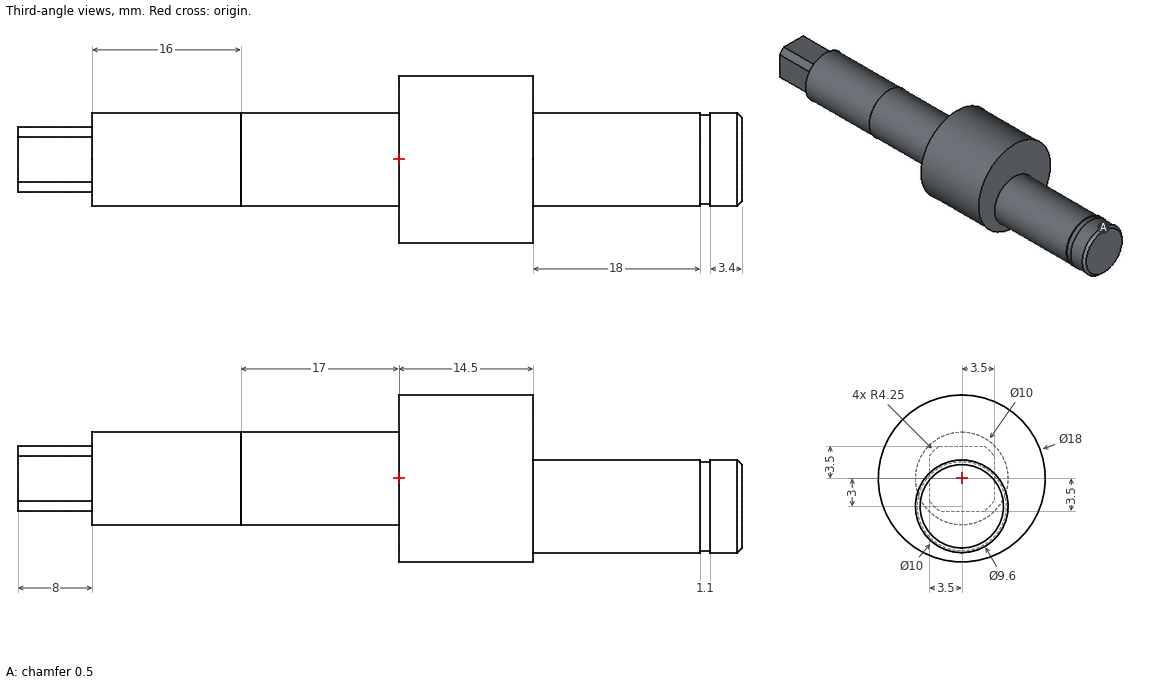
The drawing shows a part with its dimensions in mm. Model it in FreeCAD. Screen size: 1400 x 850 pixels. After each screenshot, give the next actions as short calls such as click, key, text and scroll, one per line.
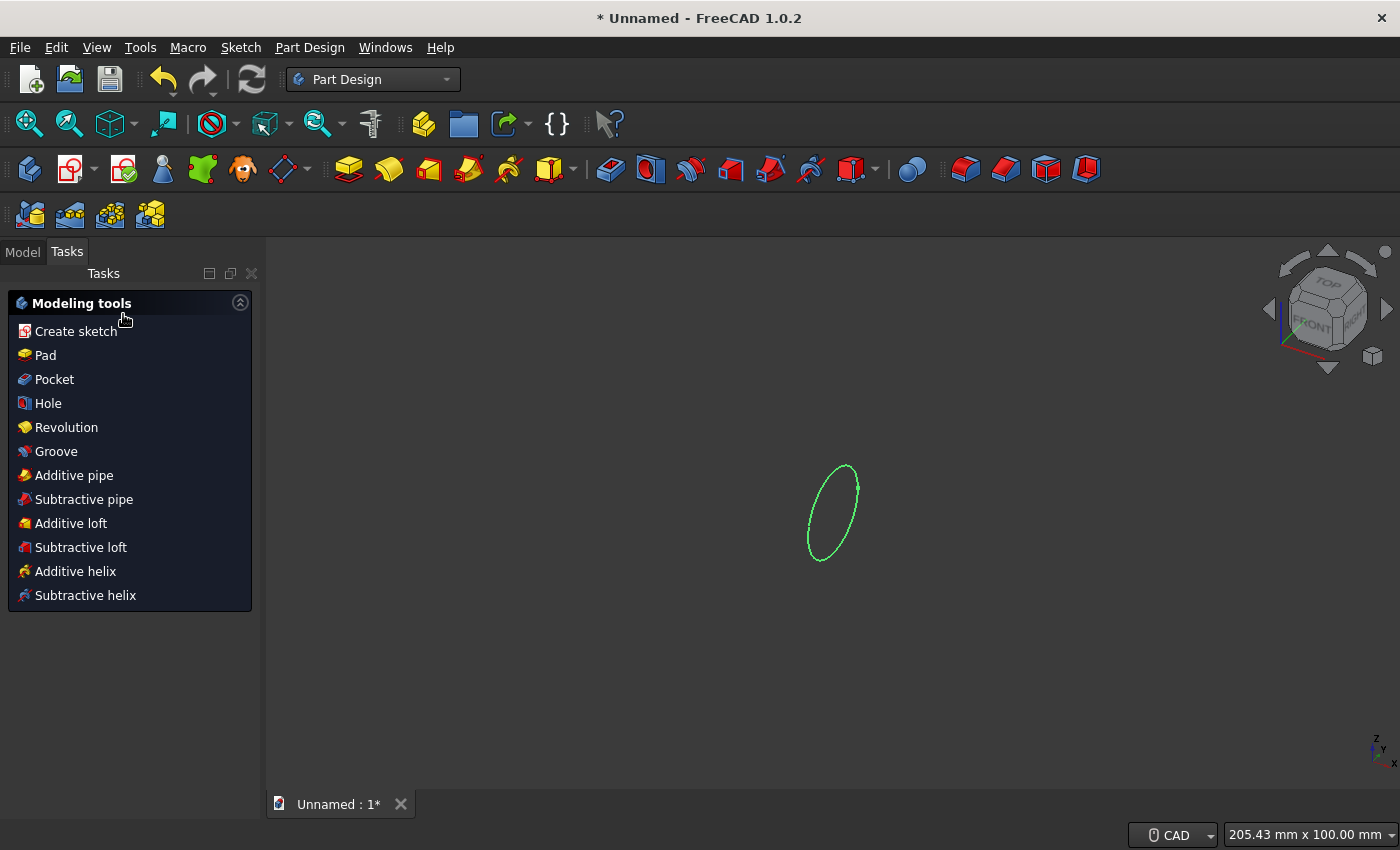
click(350, 170)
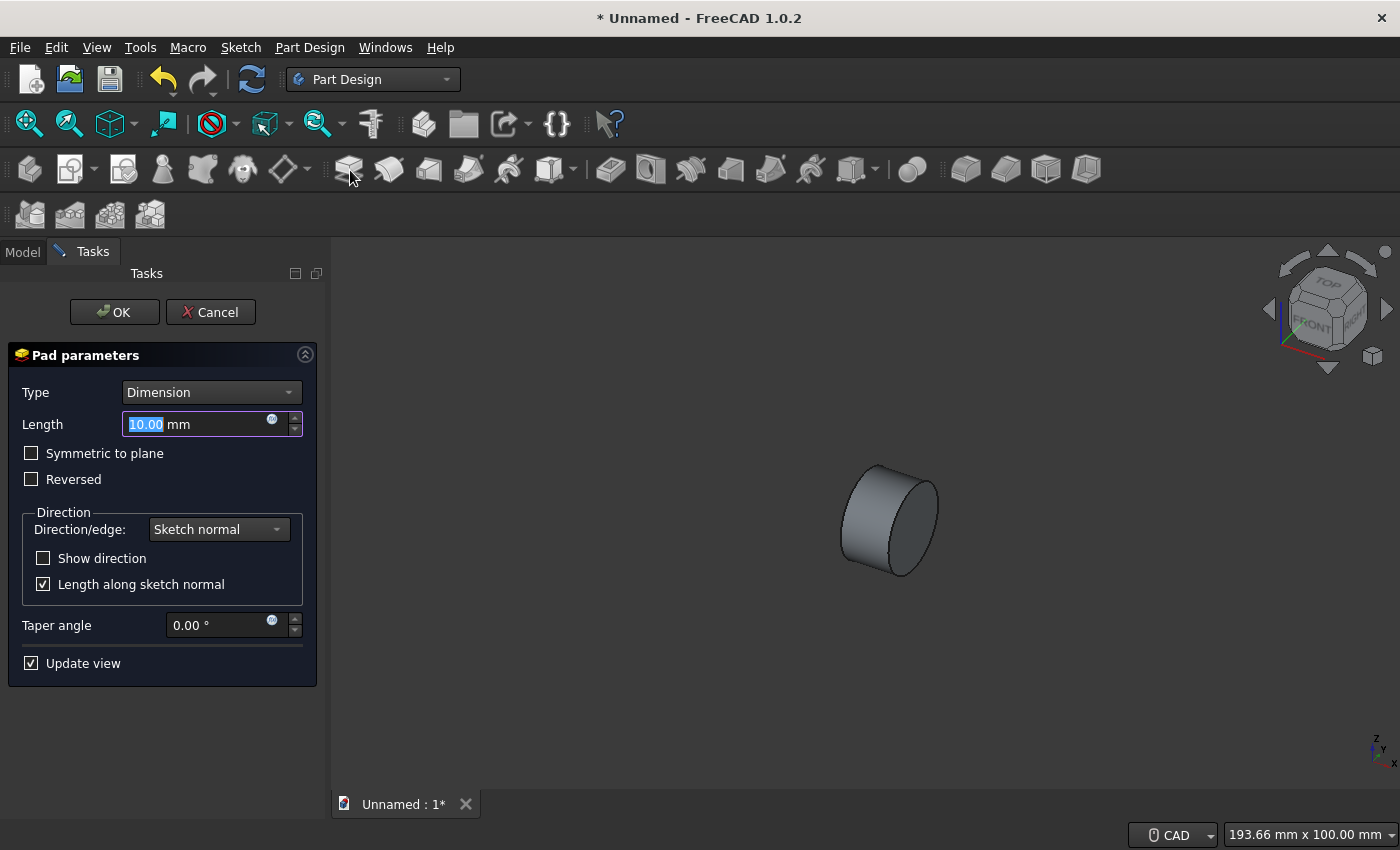
text(14.5)
key(Tab)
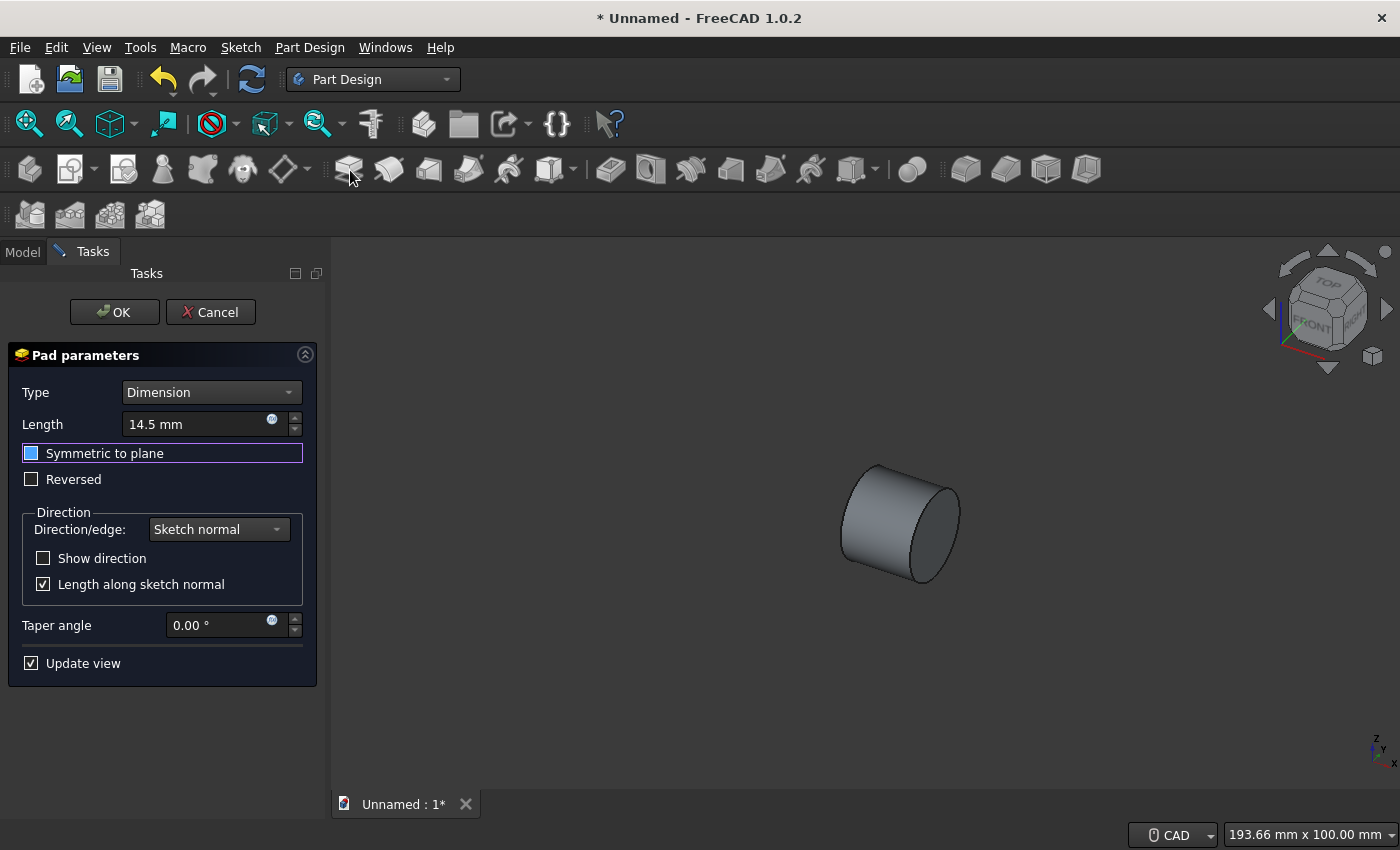
click(115, 312)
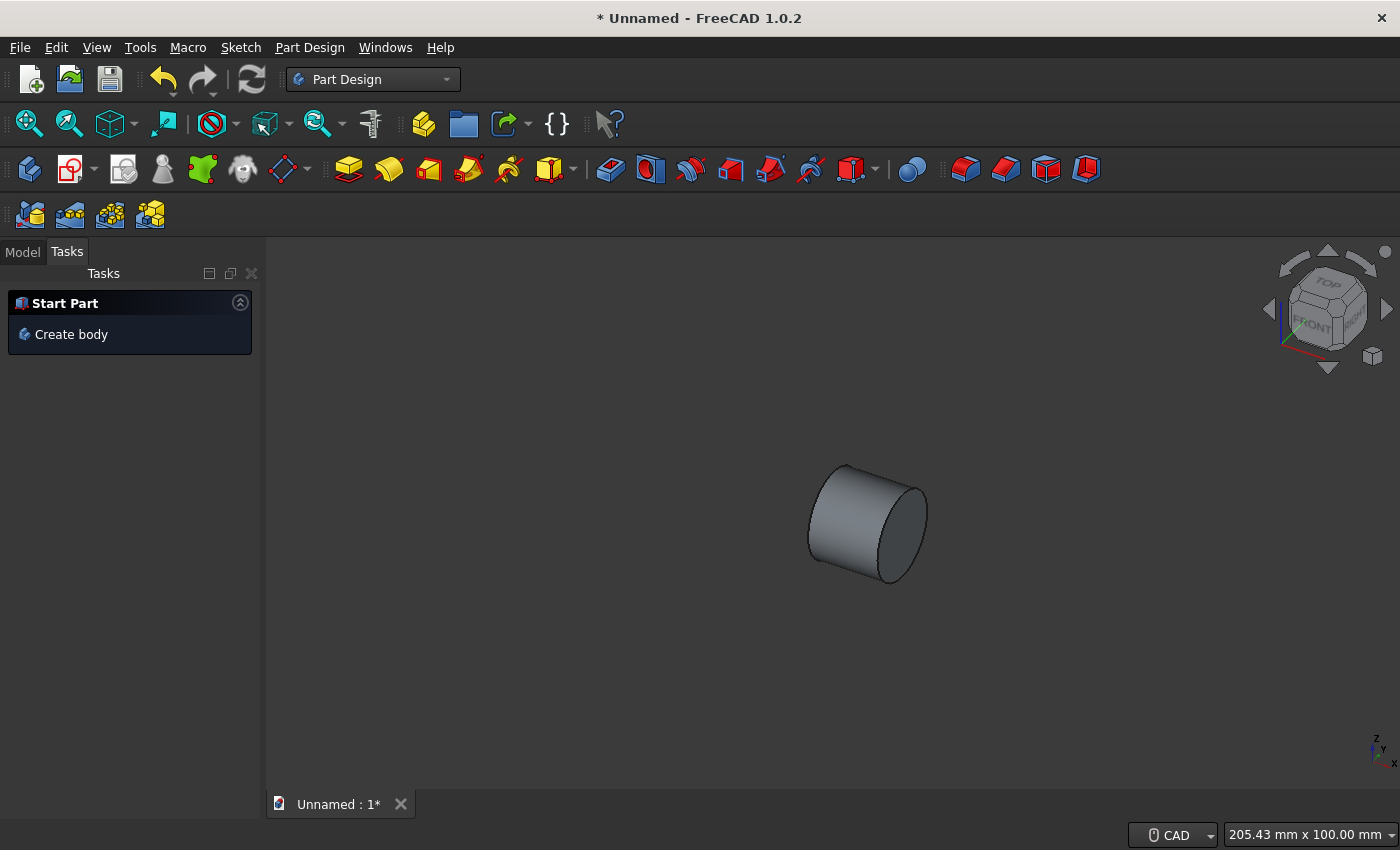
click(30, 124)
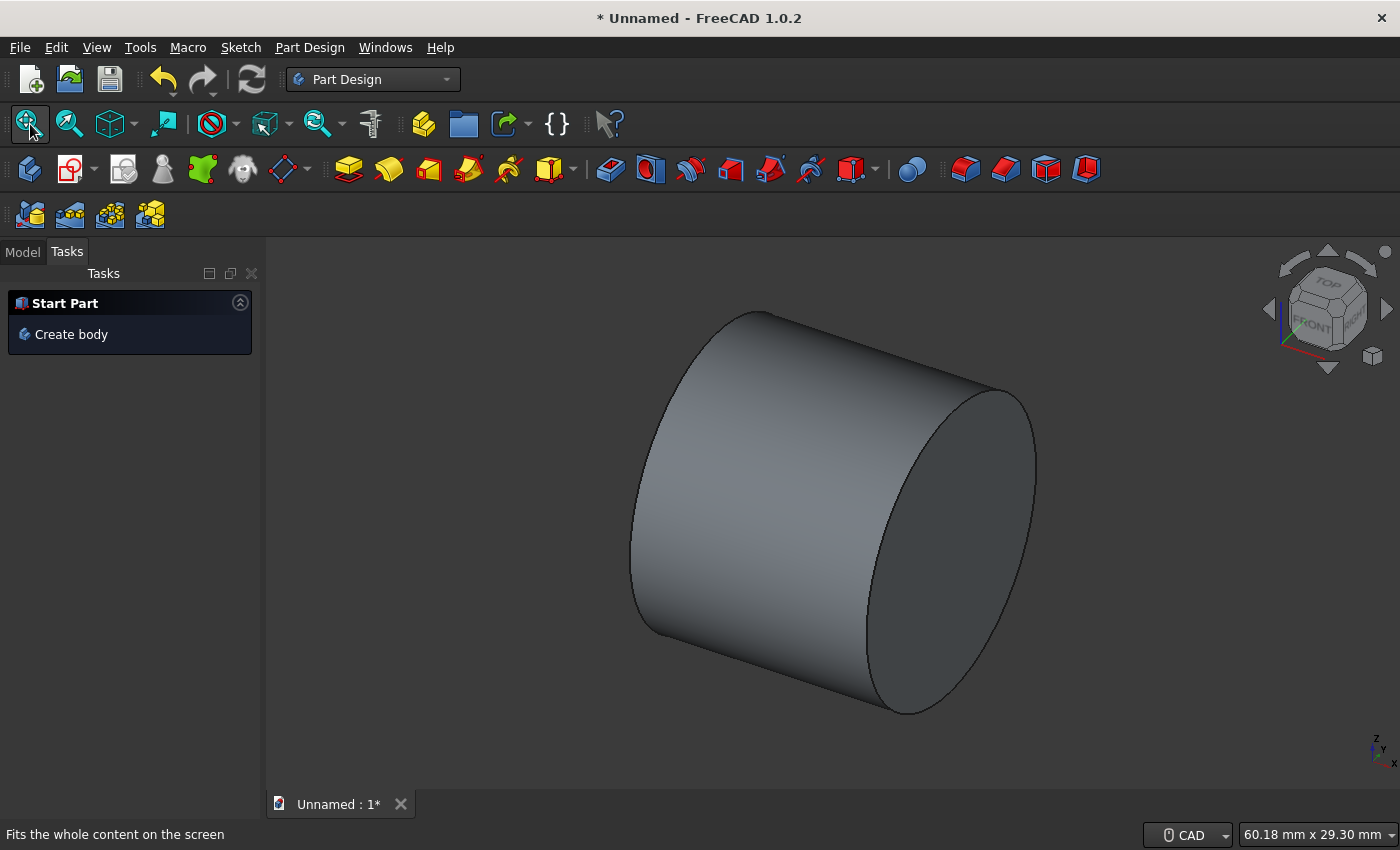
click(951, 551)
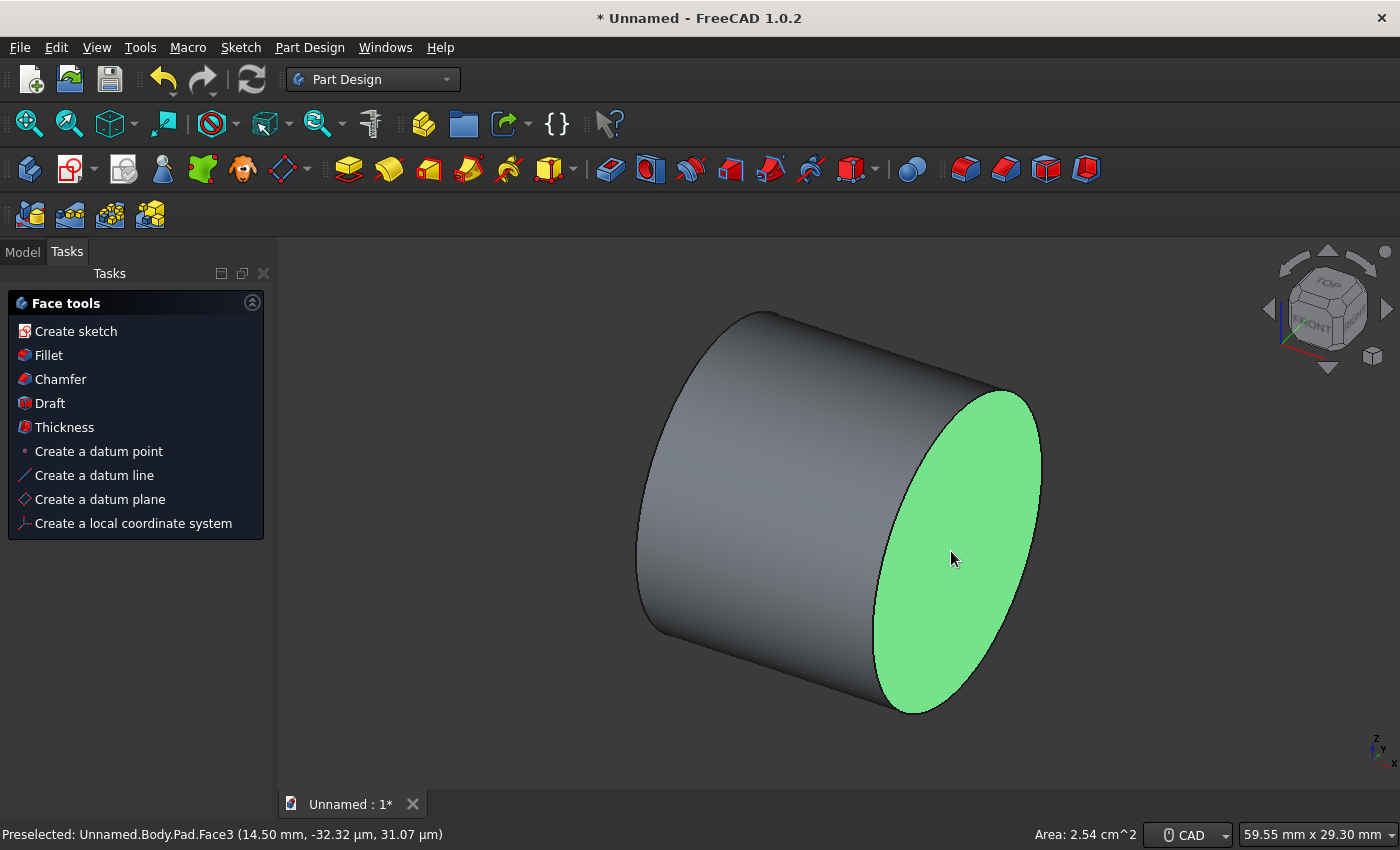
click(70, 170)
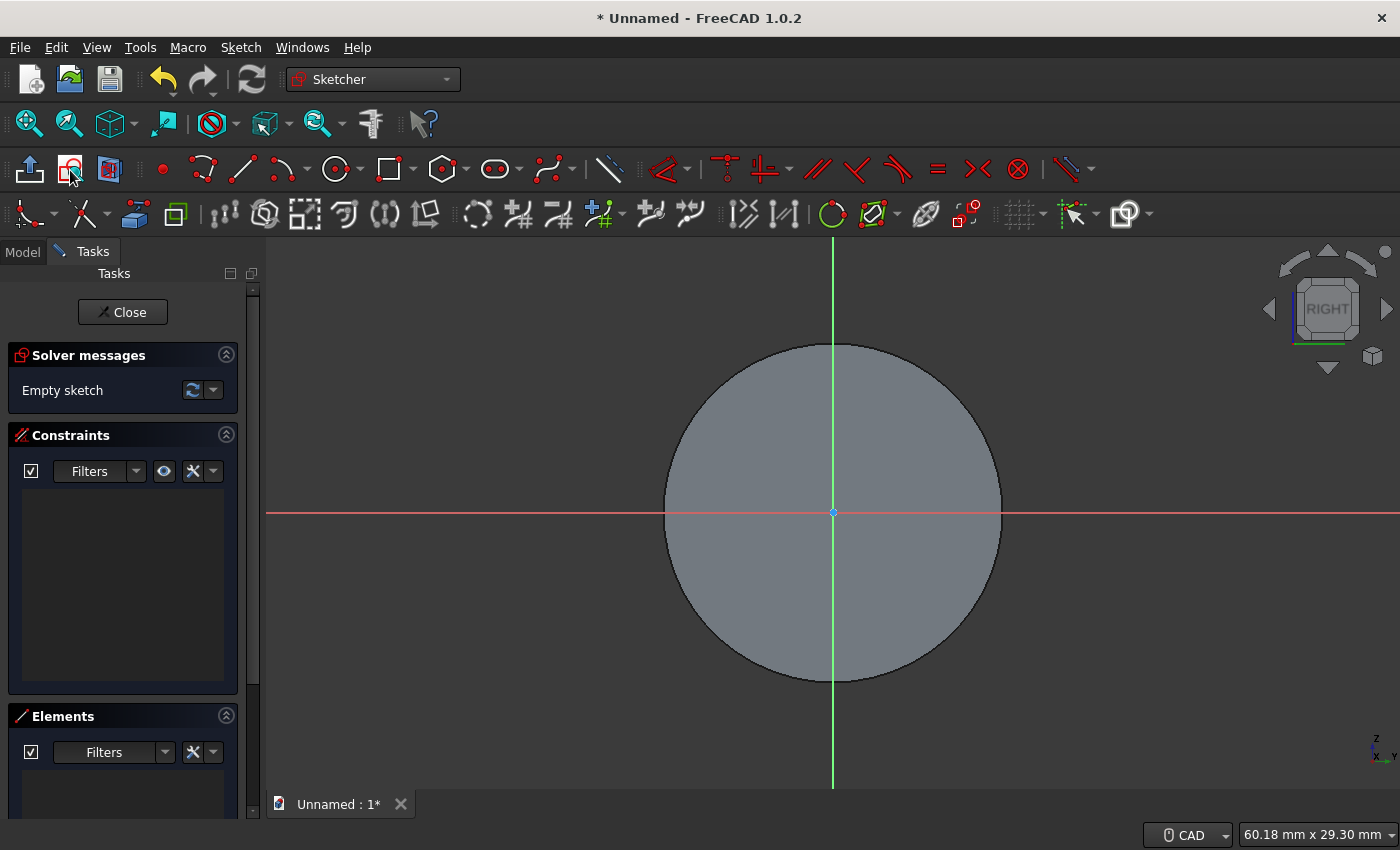
scroll(916, 638, up, 3)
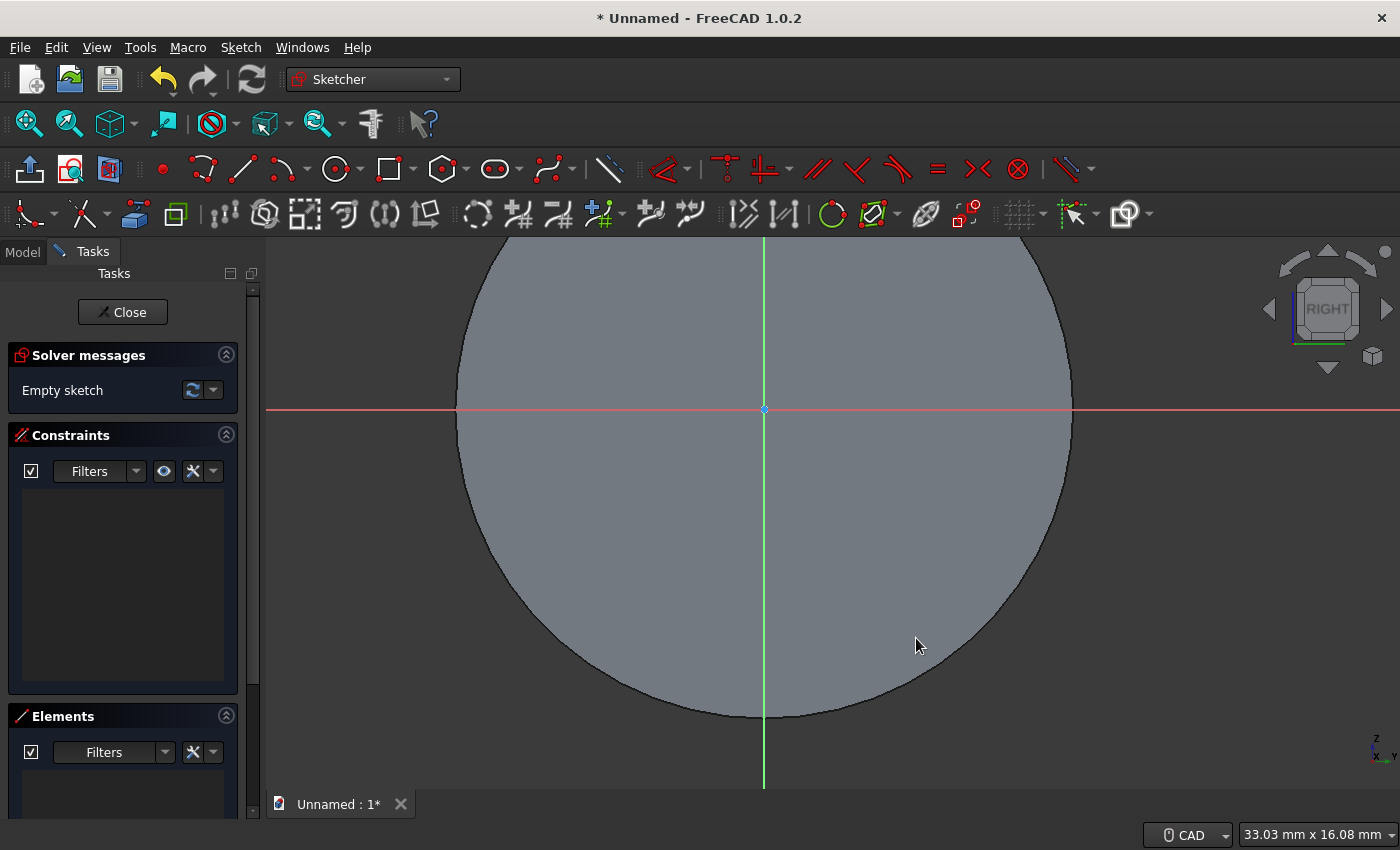
click(336, 170)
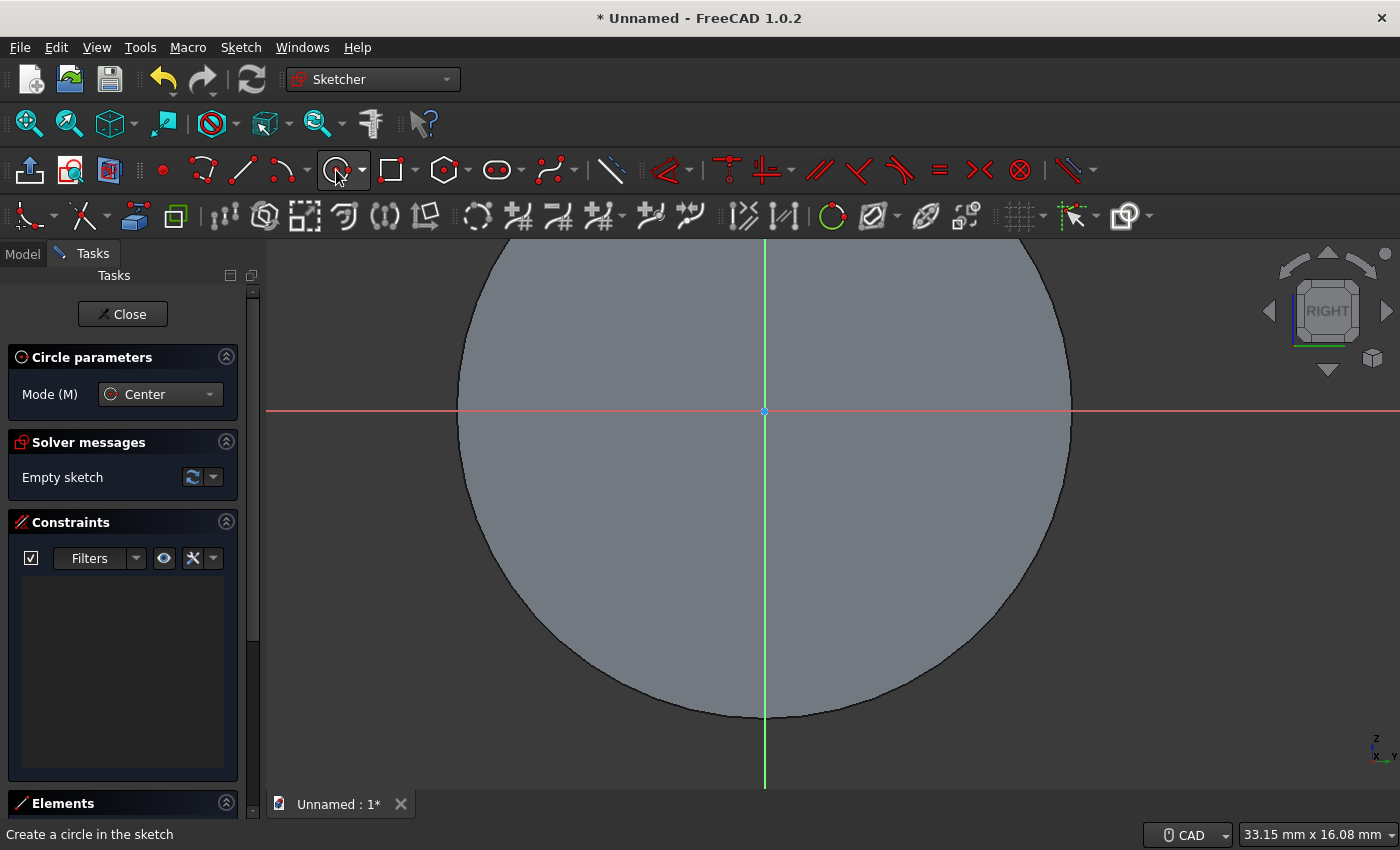
click(765, 514)
move(885, 393)